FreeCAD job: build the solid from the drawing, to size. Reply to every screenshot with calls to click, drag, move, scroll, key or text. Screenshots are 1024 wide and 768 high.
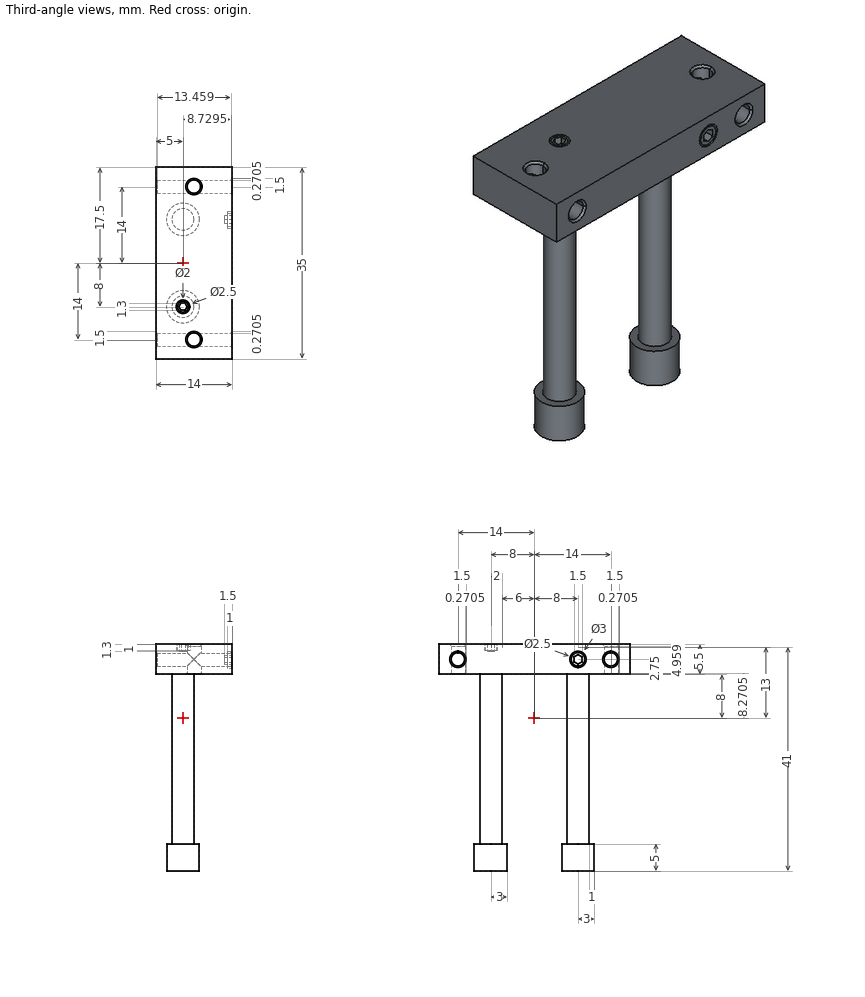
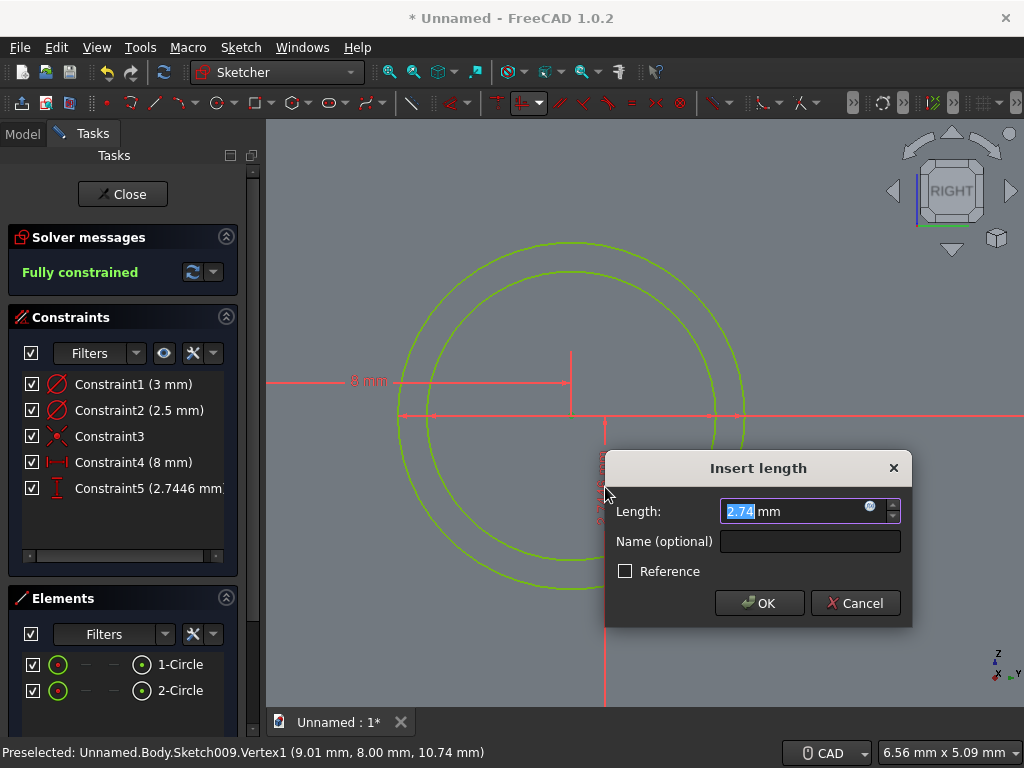
text(2.75)
key(Return)
key(Escape)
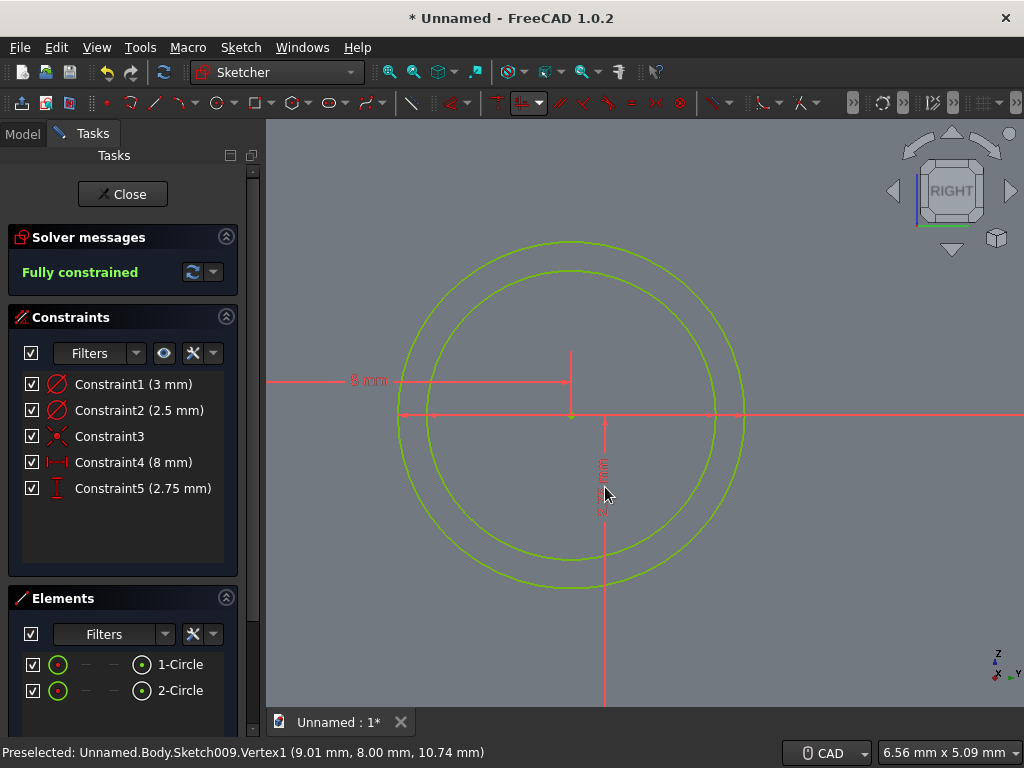
click(123, 194)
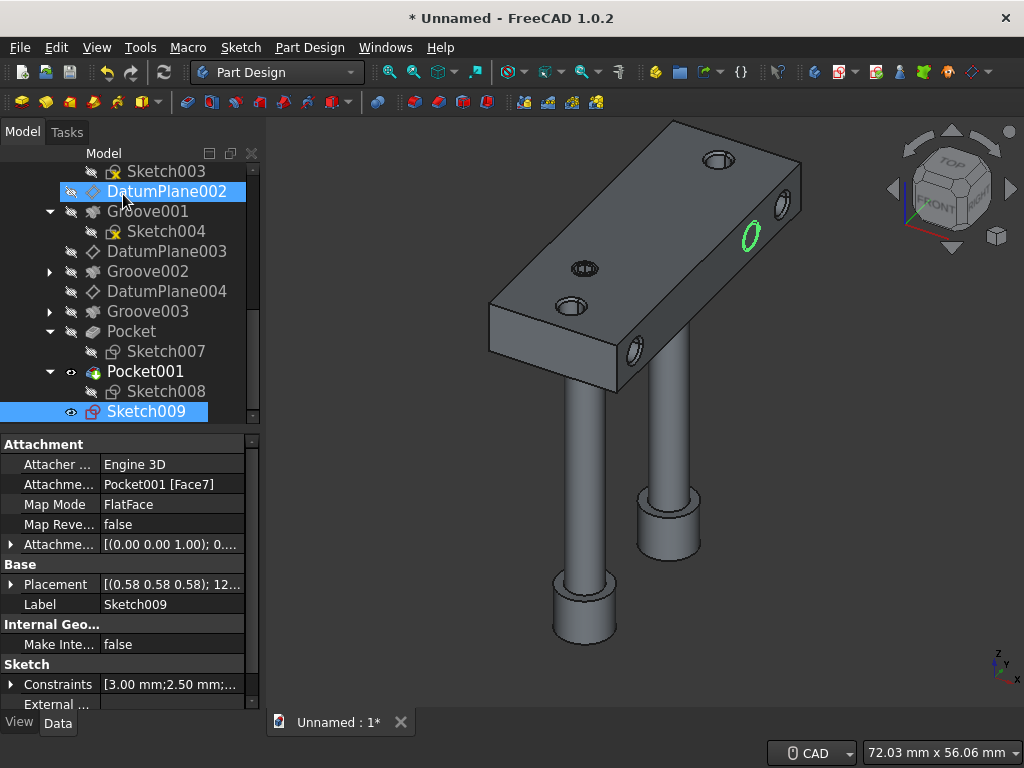
click(188, 102)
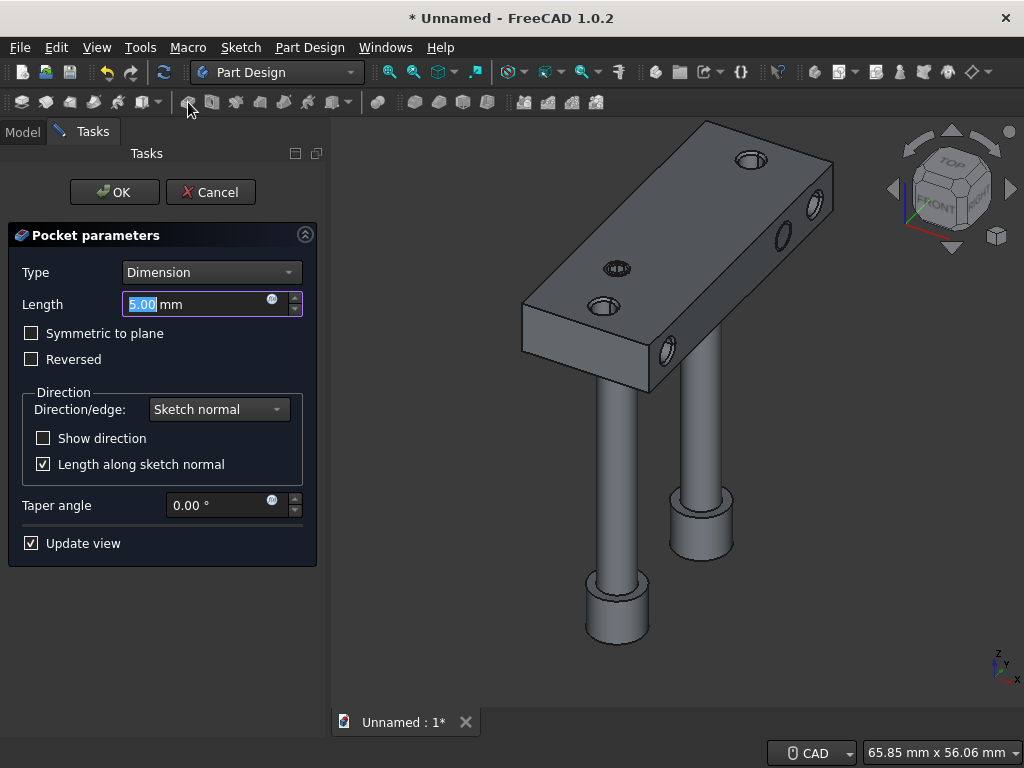
text(1)
key(Tab)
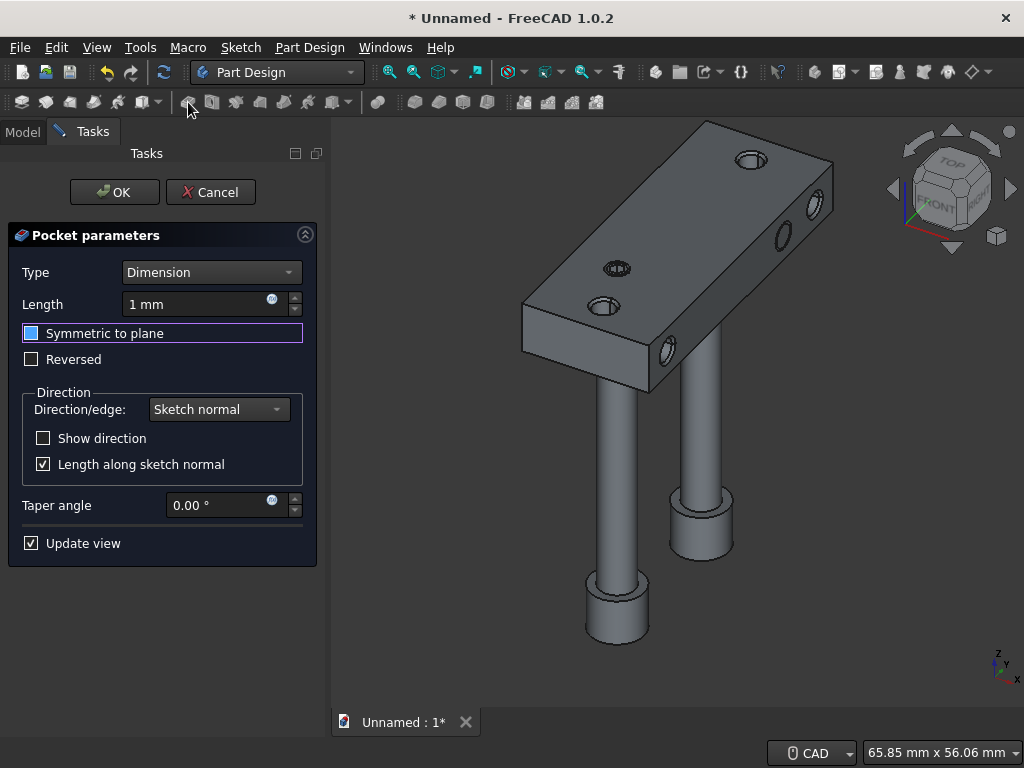
click(115, 192)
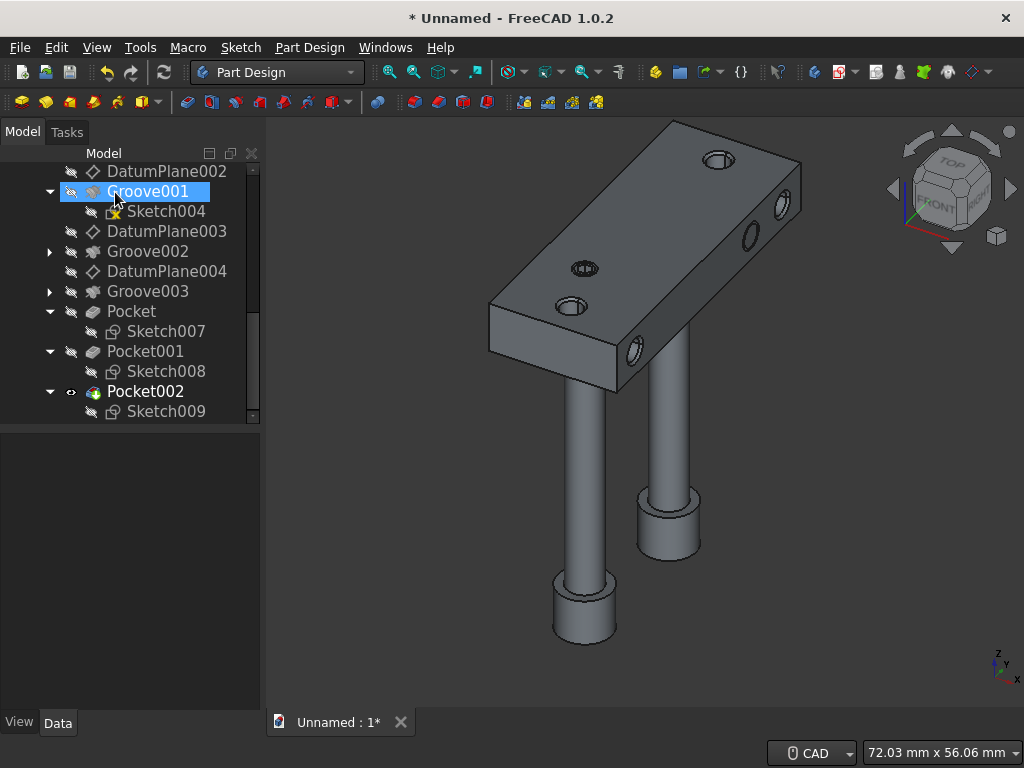
click(709, 277)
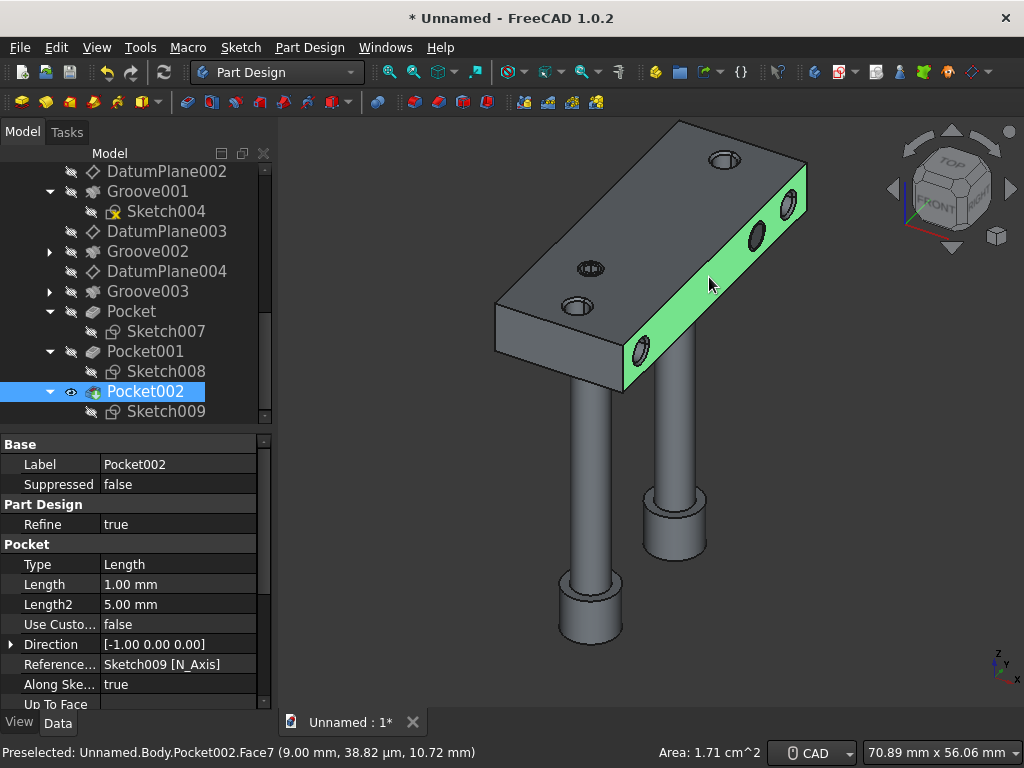
click(840, 72)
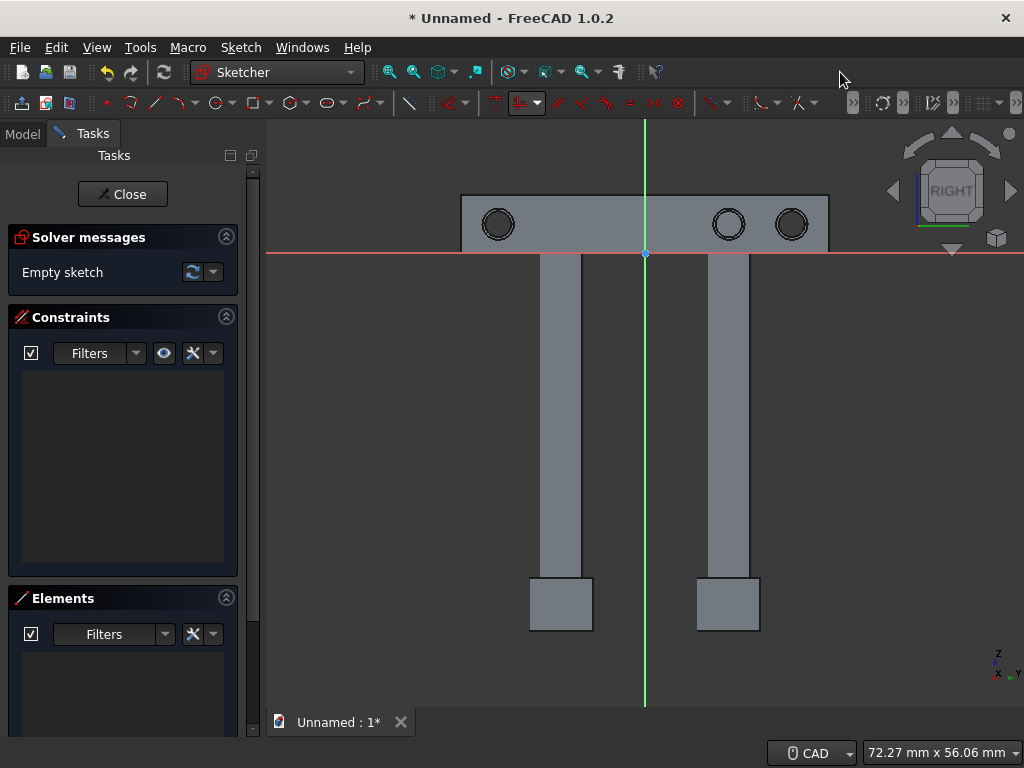
scroll(737, 214, up, 15)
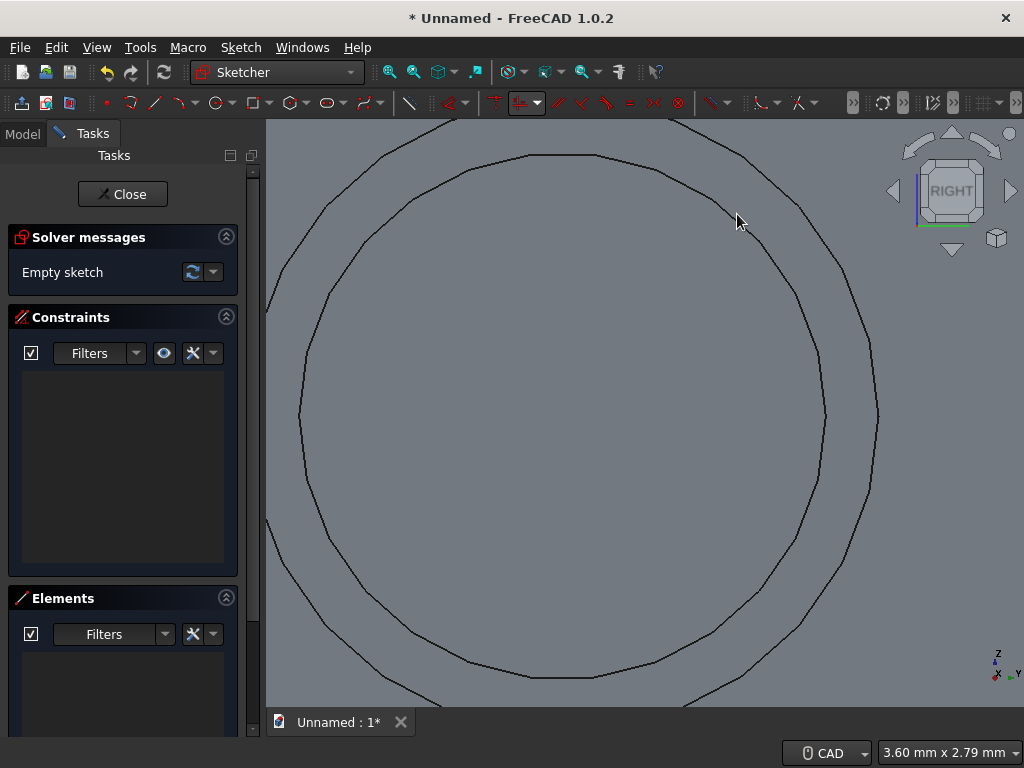
click(290, 104)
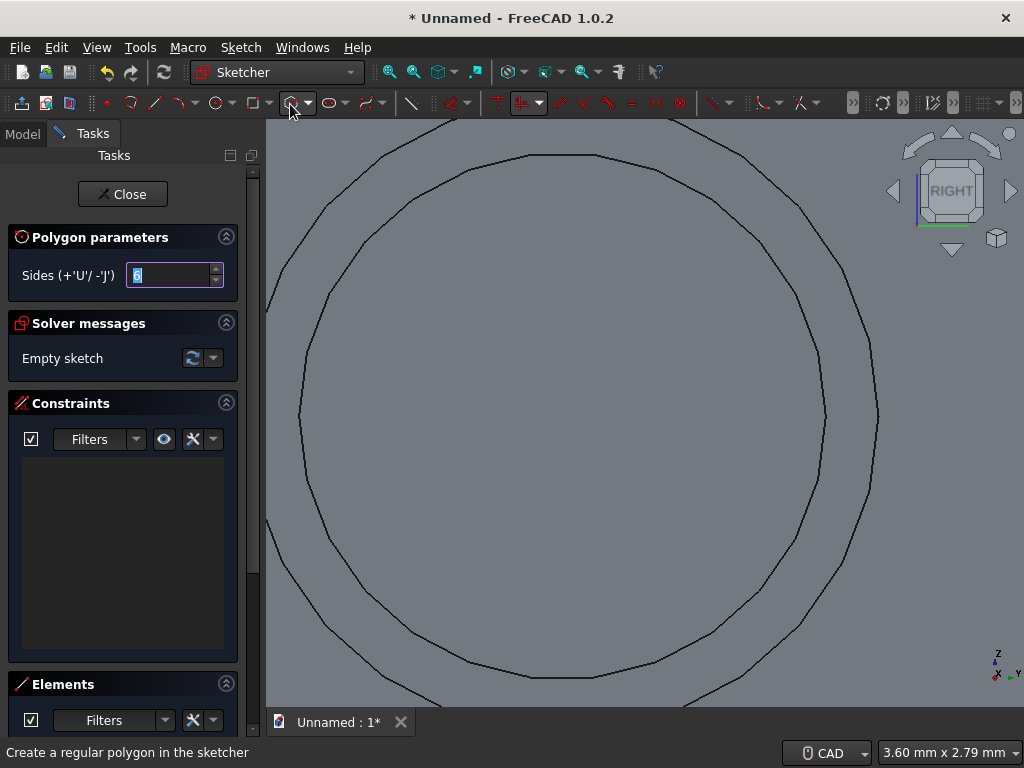
click(562, 416)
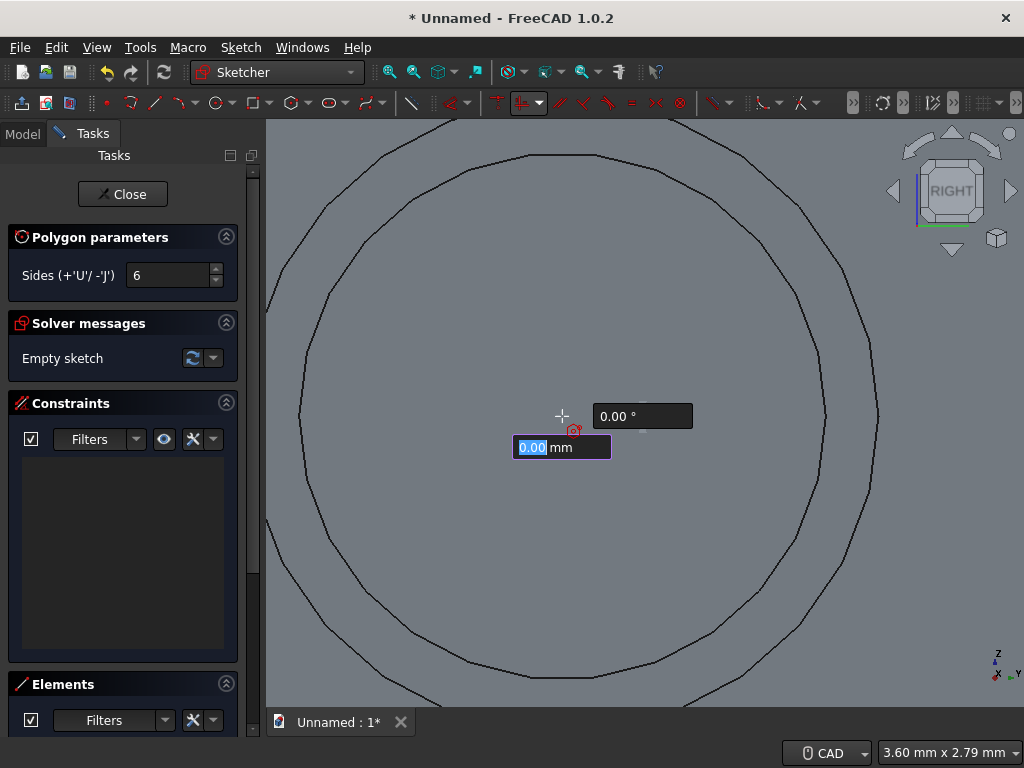
click(562, 234)
right_click(562, 234)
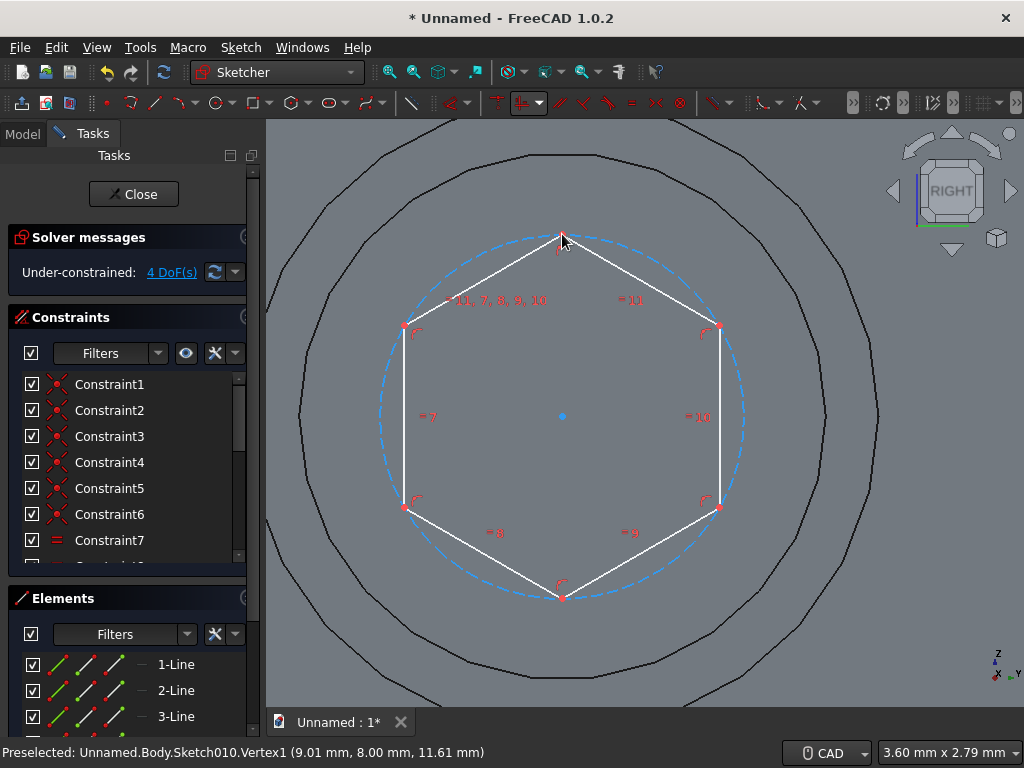
click(404, 381)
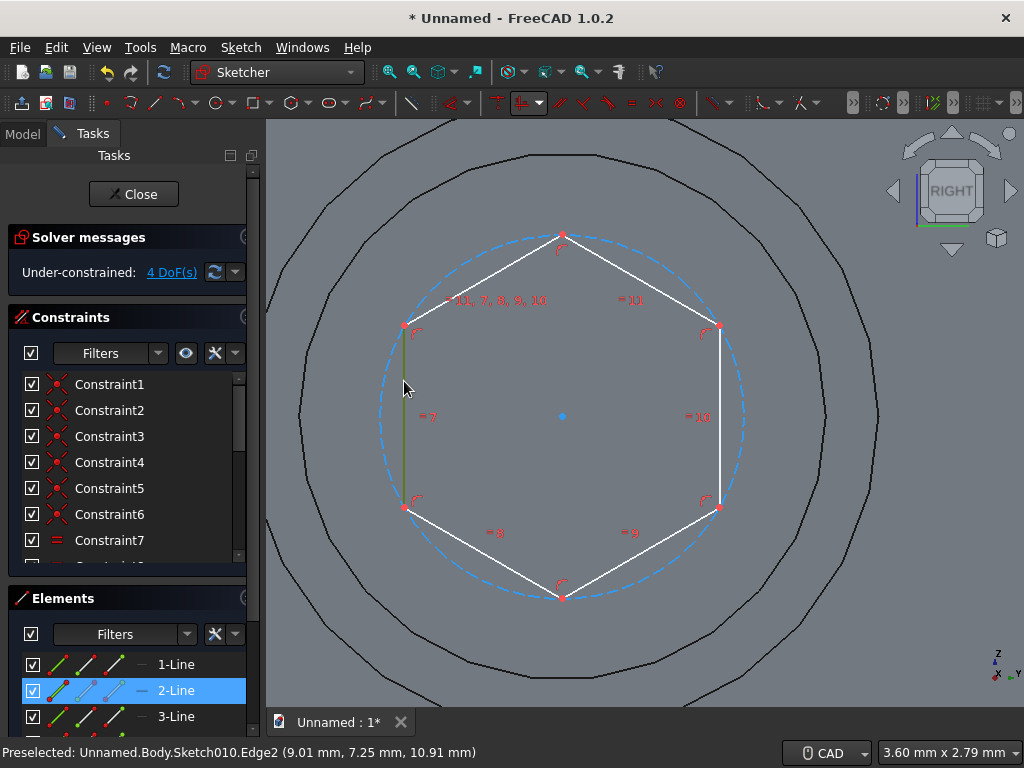
key(v)